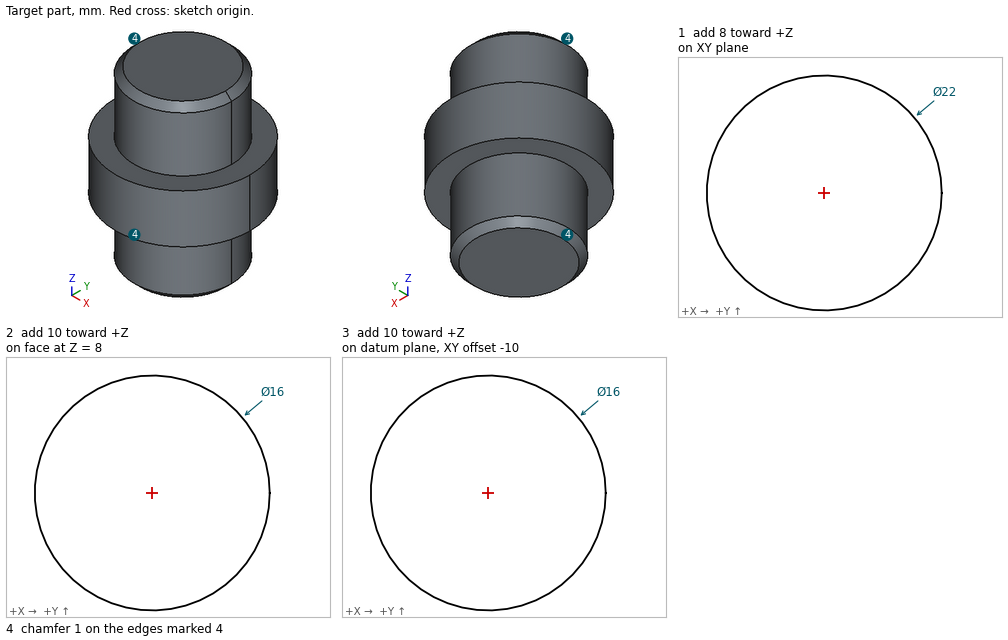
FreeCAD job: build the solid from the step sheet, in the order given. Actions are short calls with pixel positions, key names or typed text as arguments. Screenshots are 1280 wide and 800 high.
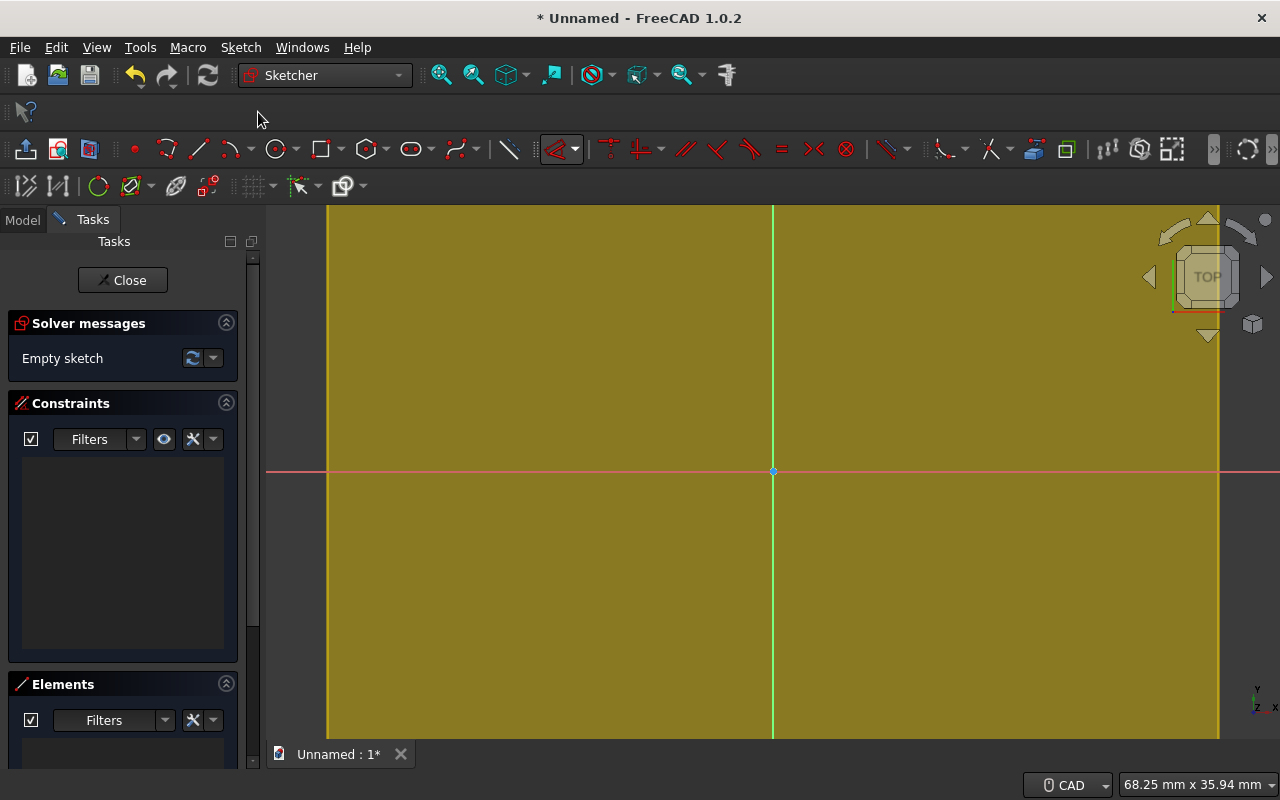
scroll(912, 472, up, 2)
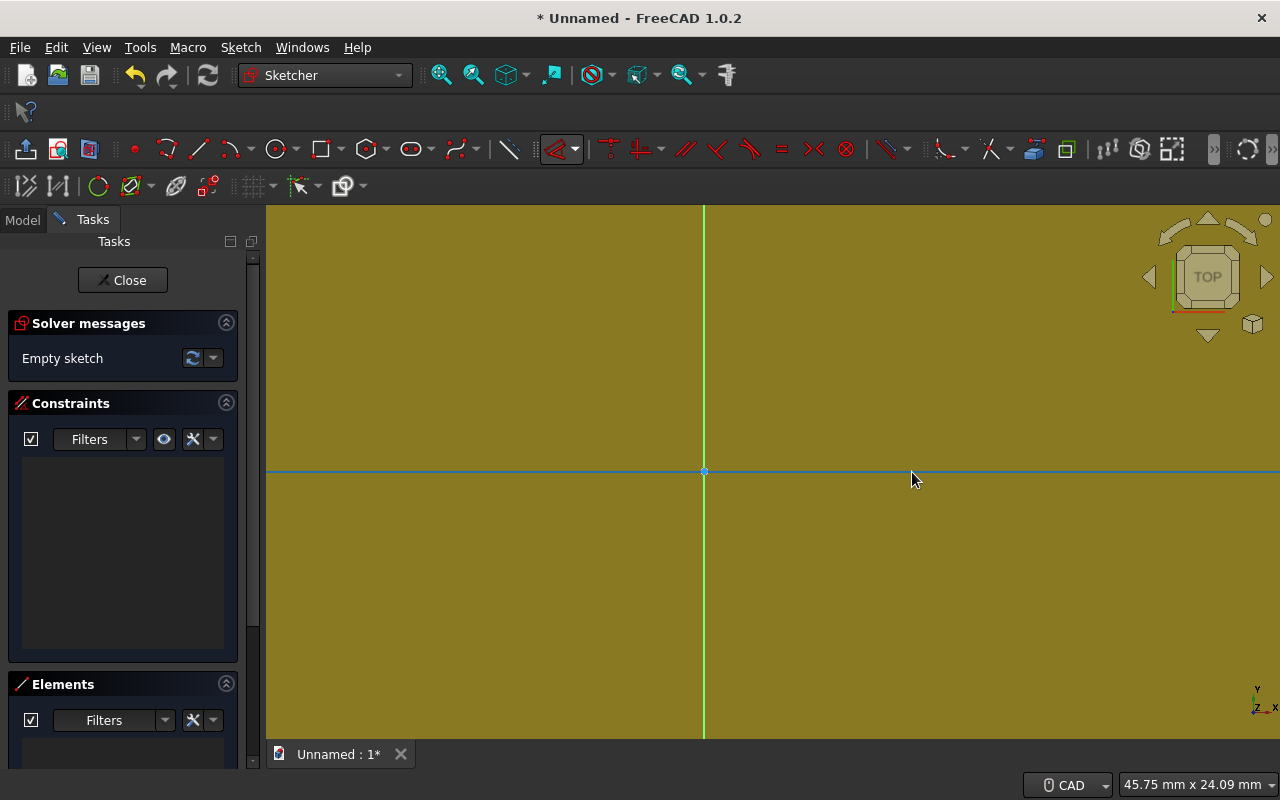
click(276, 150)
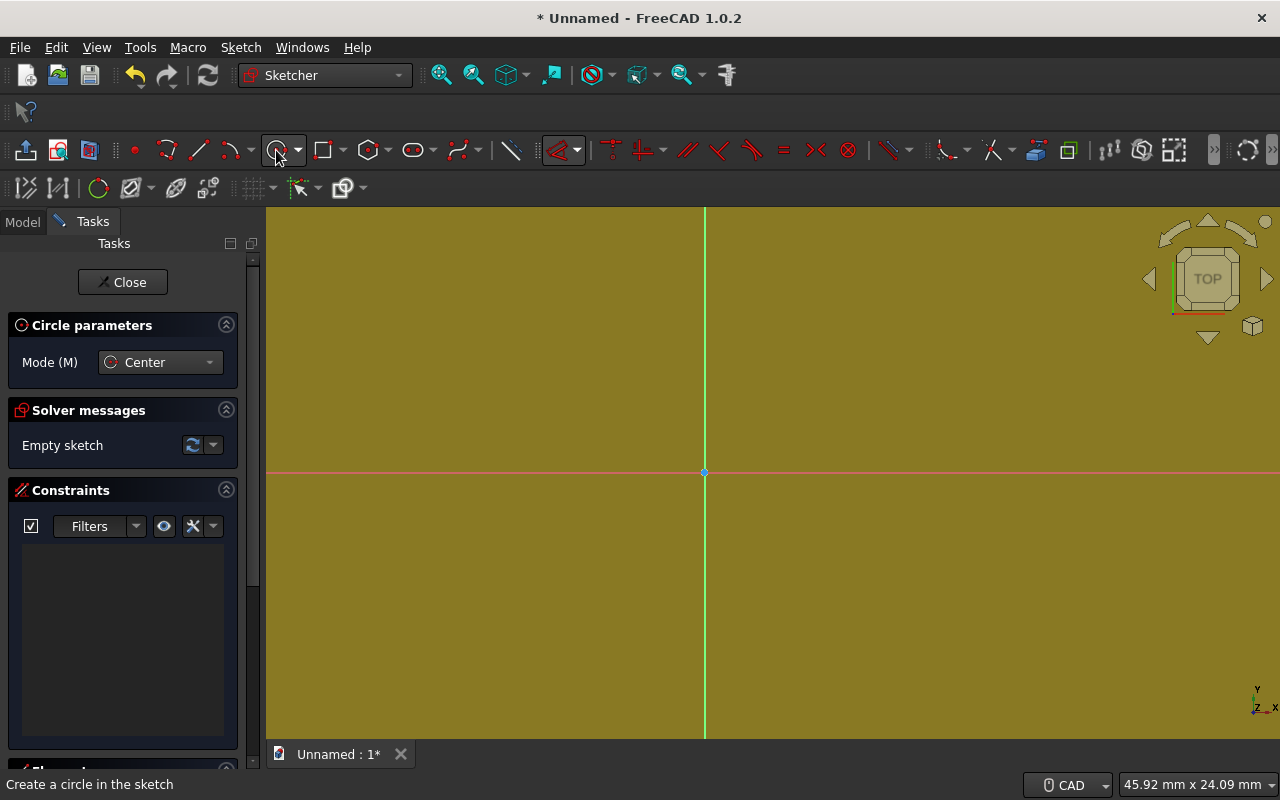
click(705, 473)
click(829, 348)
key(Escape)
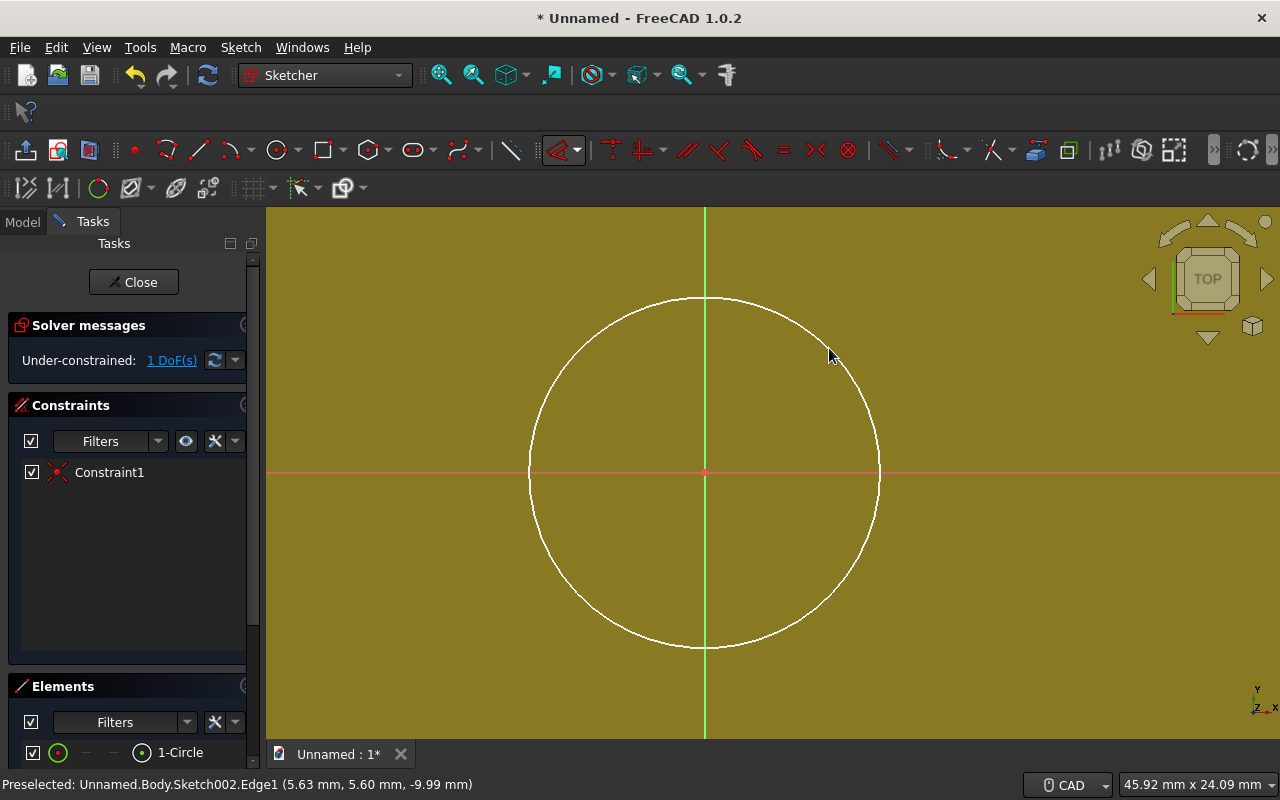
click(828, 348)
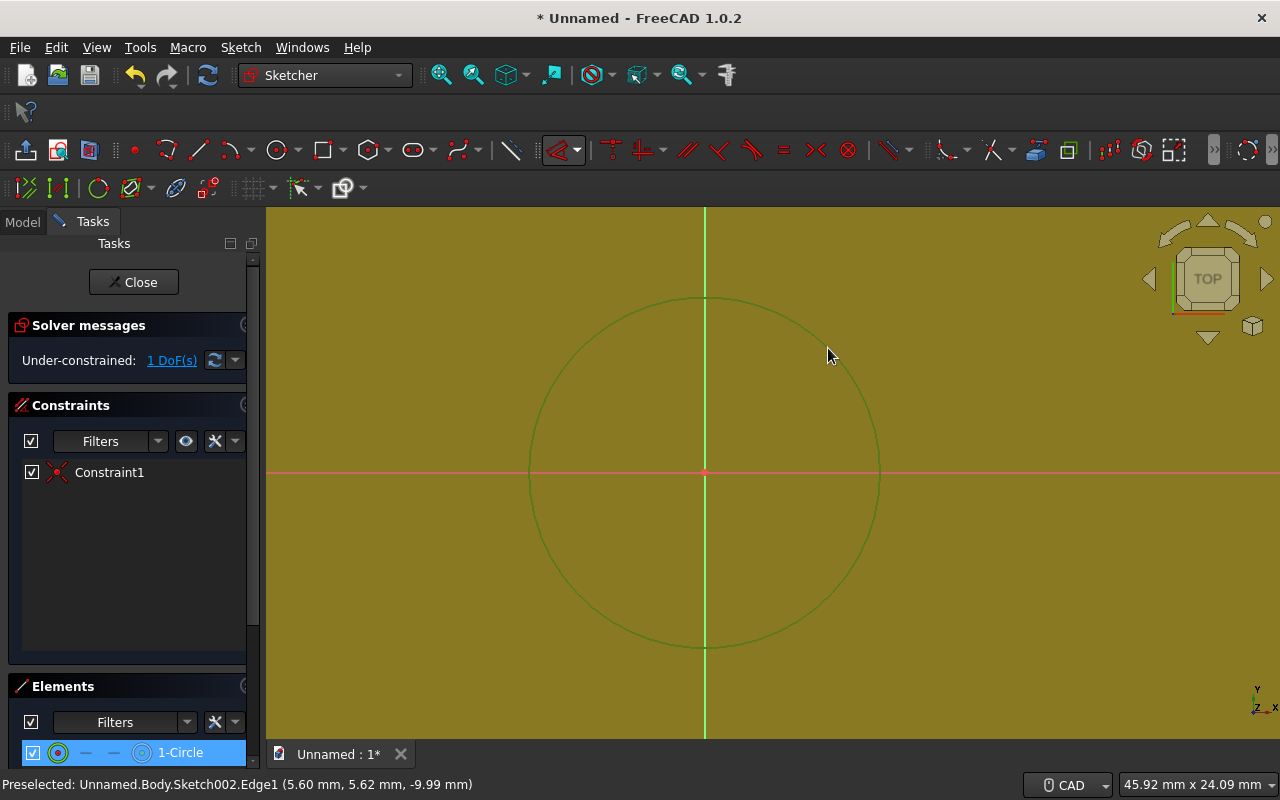
key(k)
key(o)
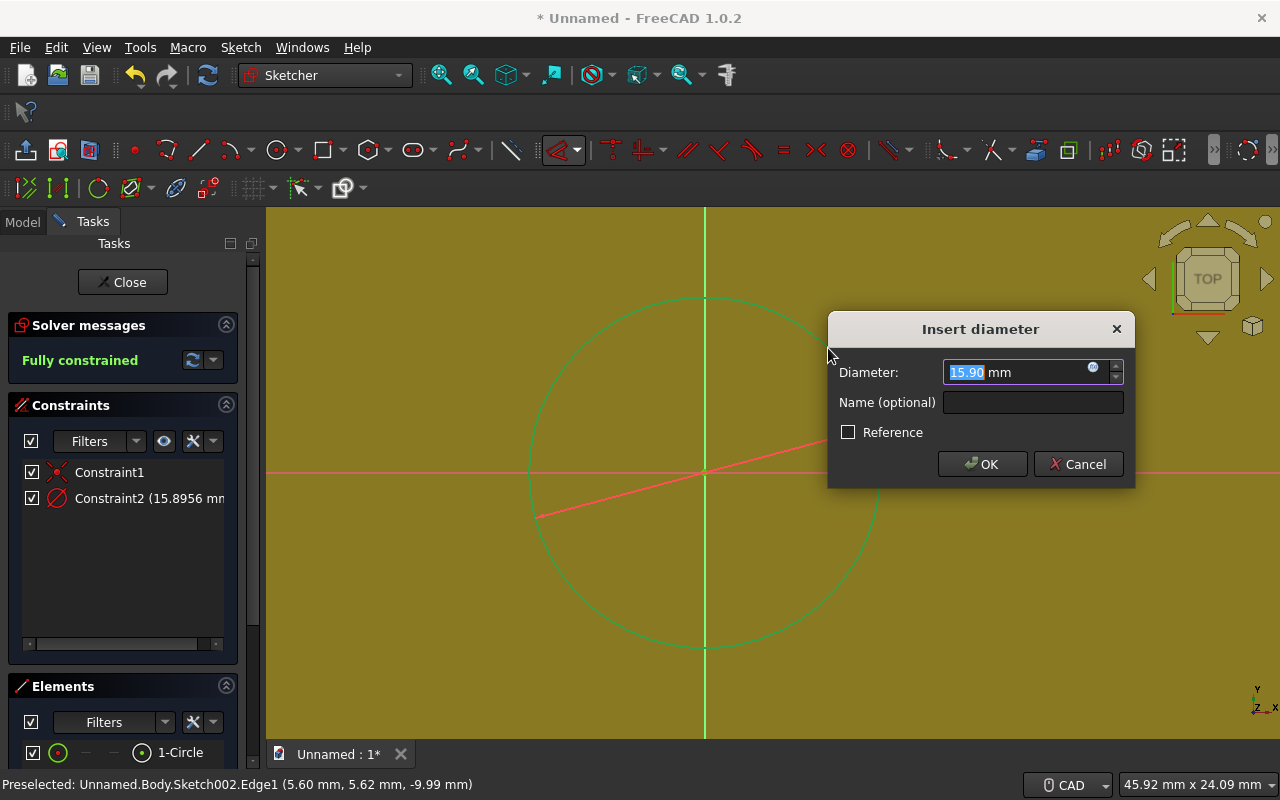
text(16)
key(Return)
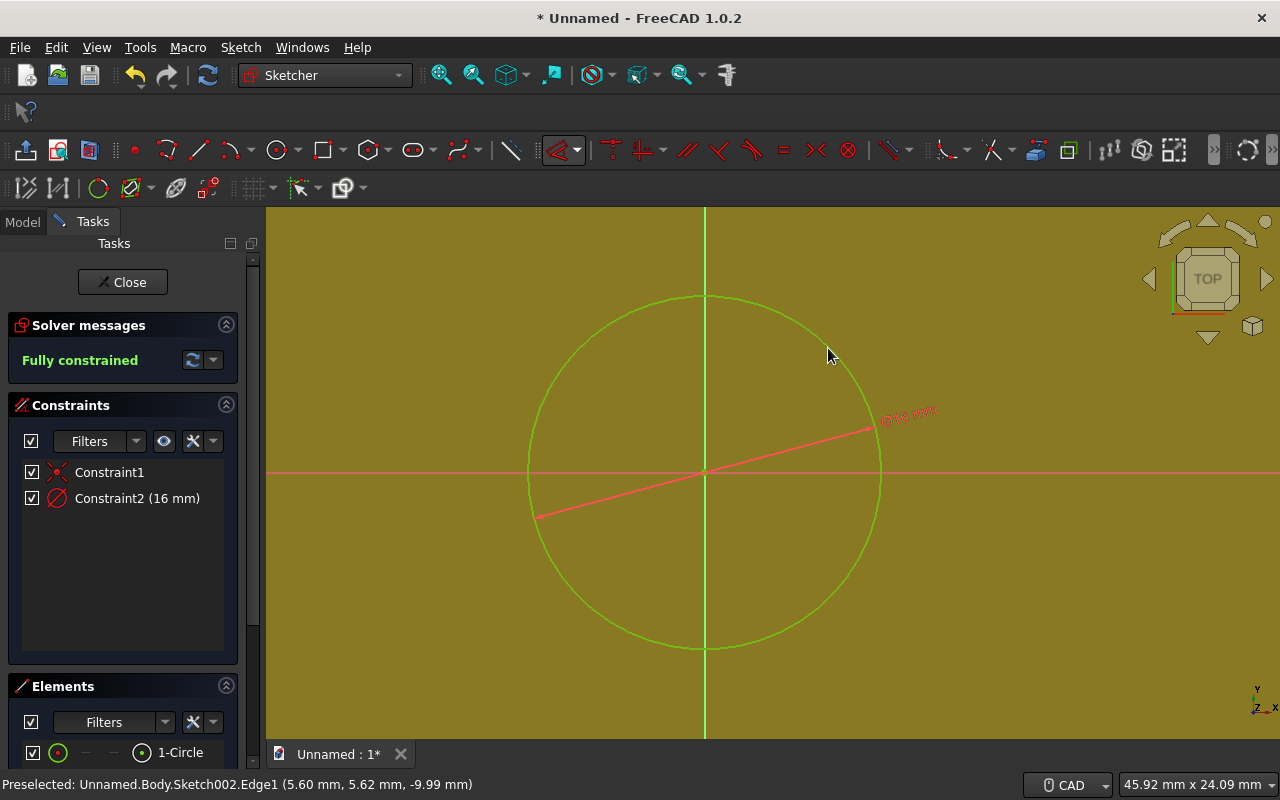
click(123, 282)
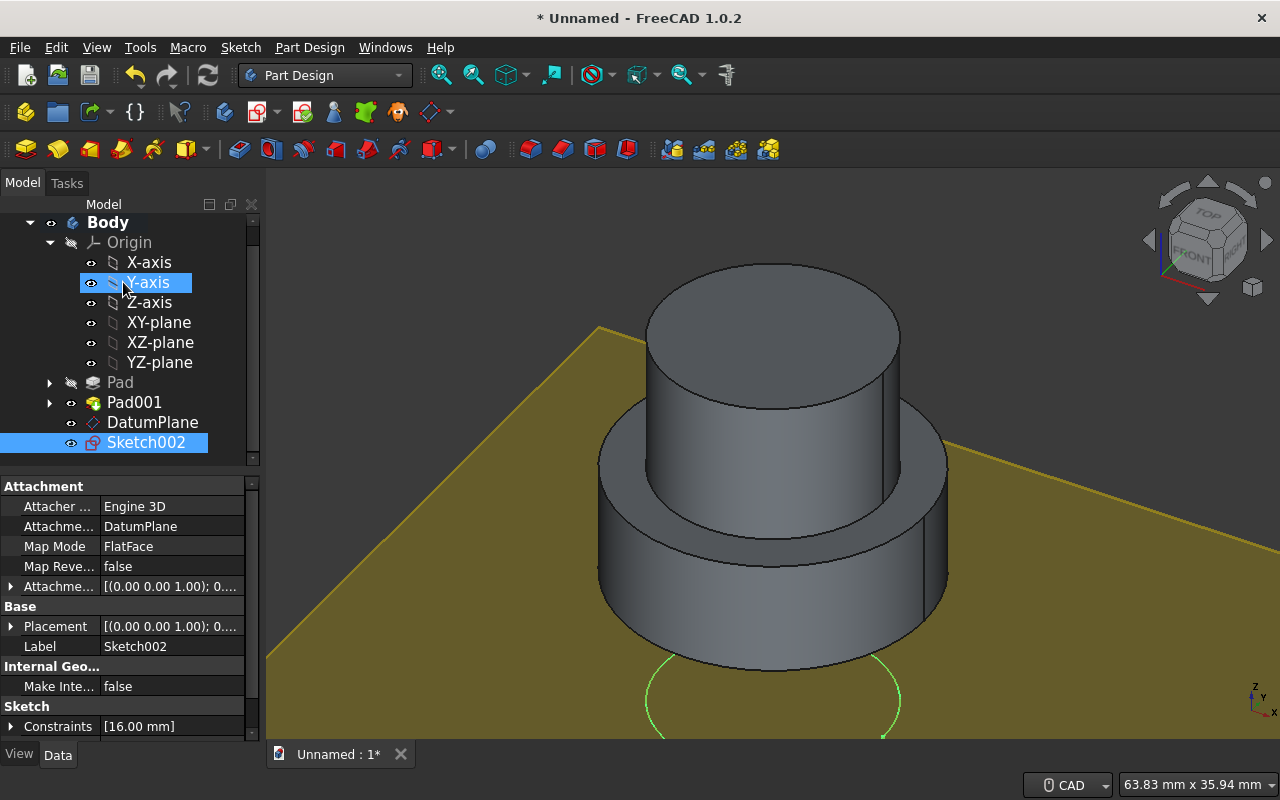
click(26, 150)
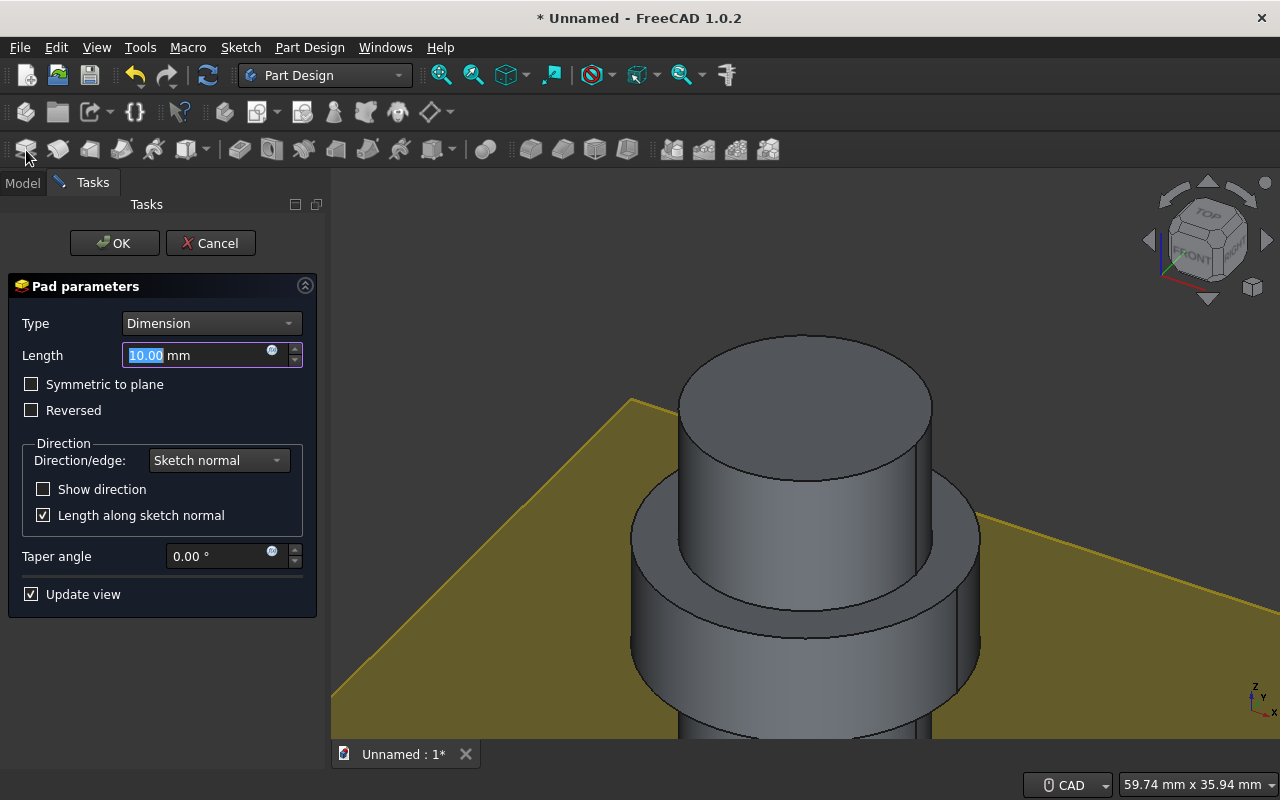
text(10)
key(Tab)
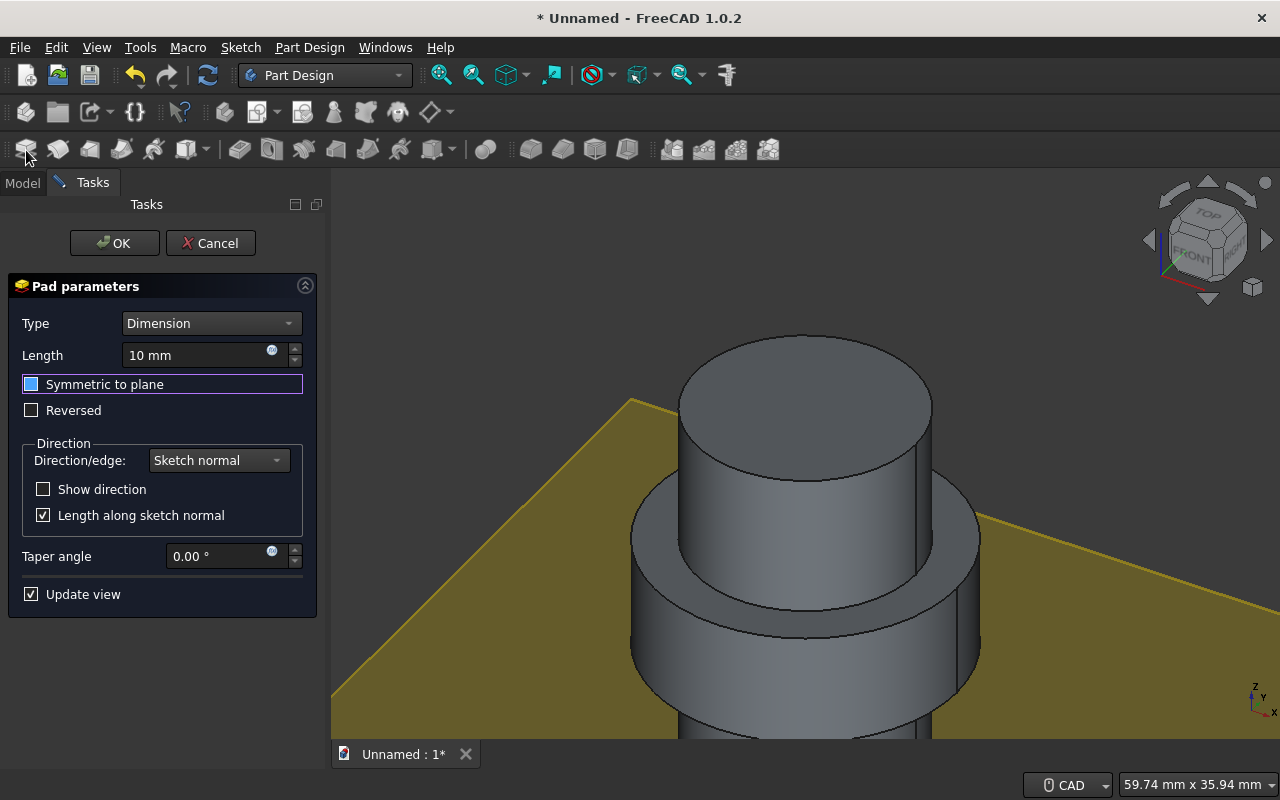
click(115, 243)